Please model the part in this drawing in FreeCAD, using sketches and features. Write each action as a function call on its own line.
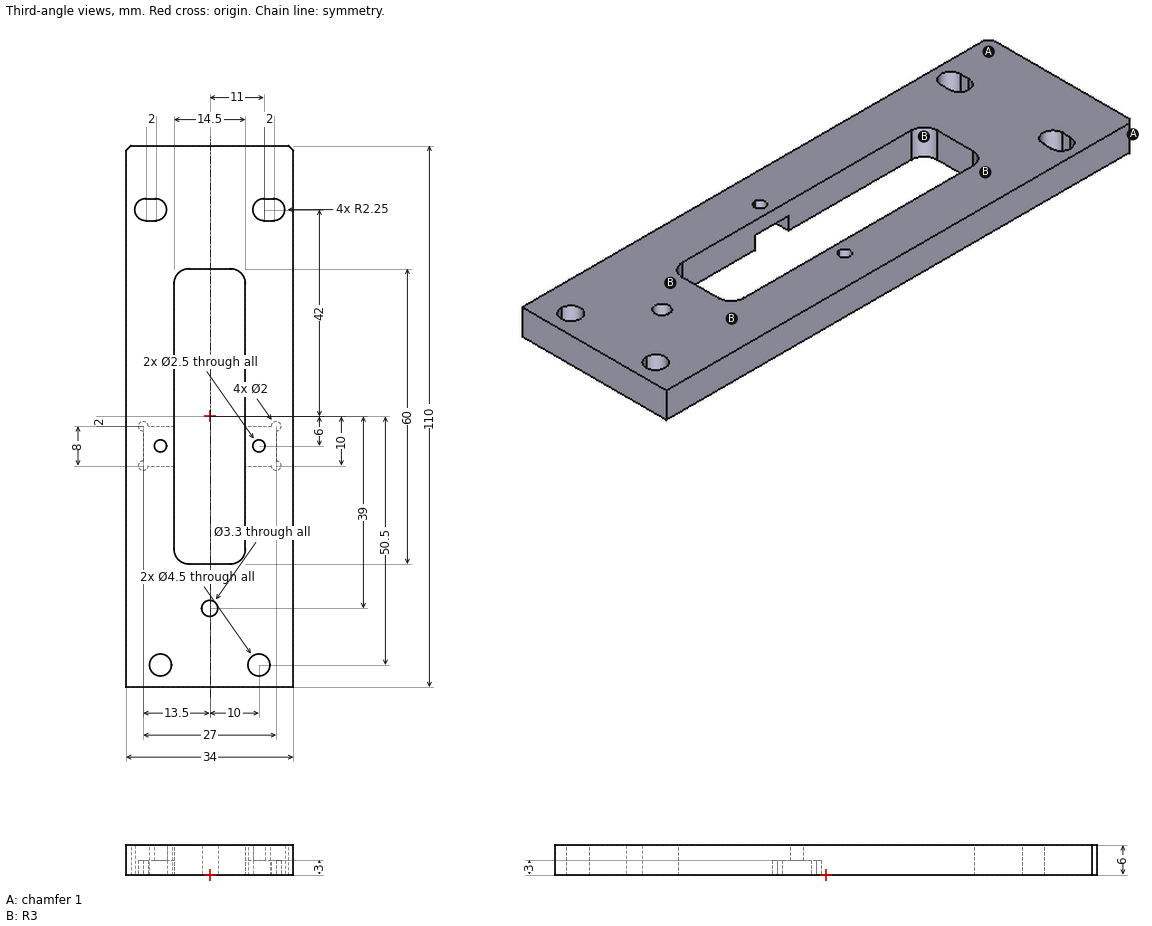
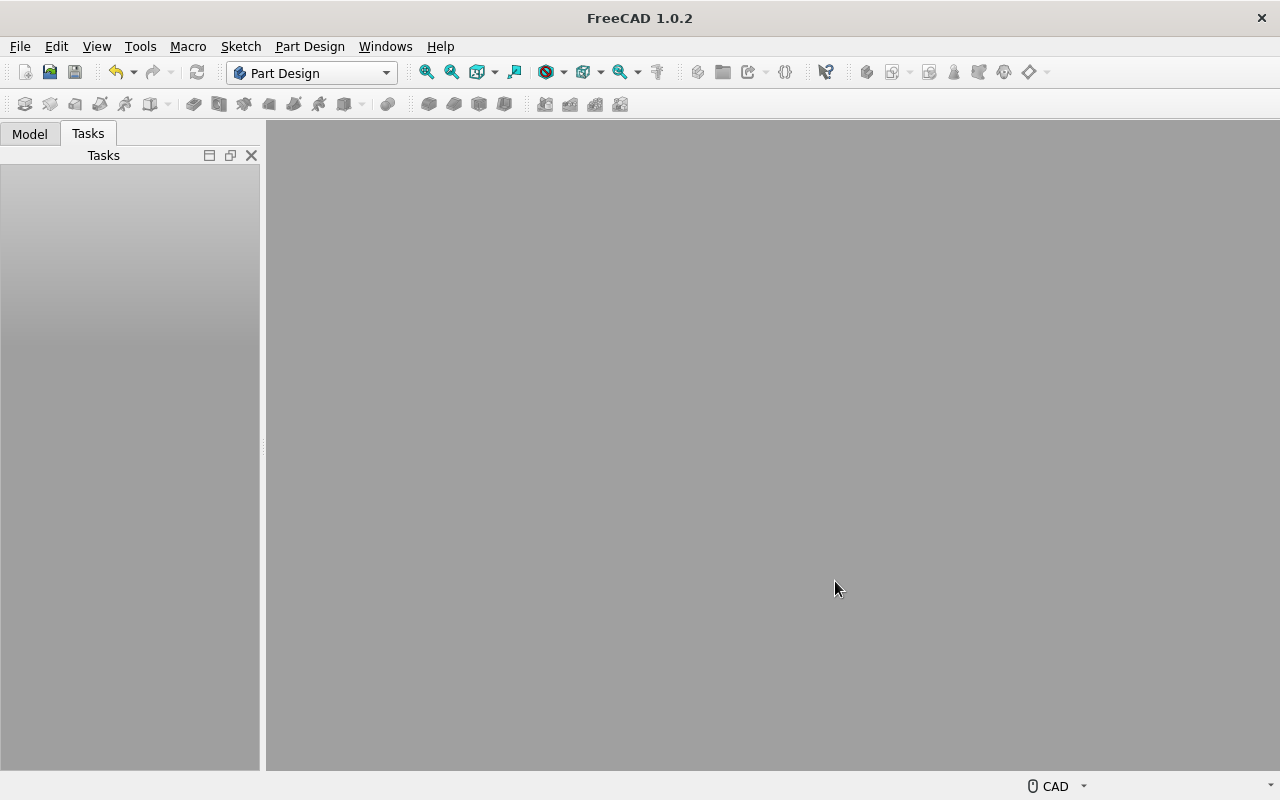
key(ctrl+n)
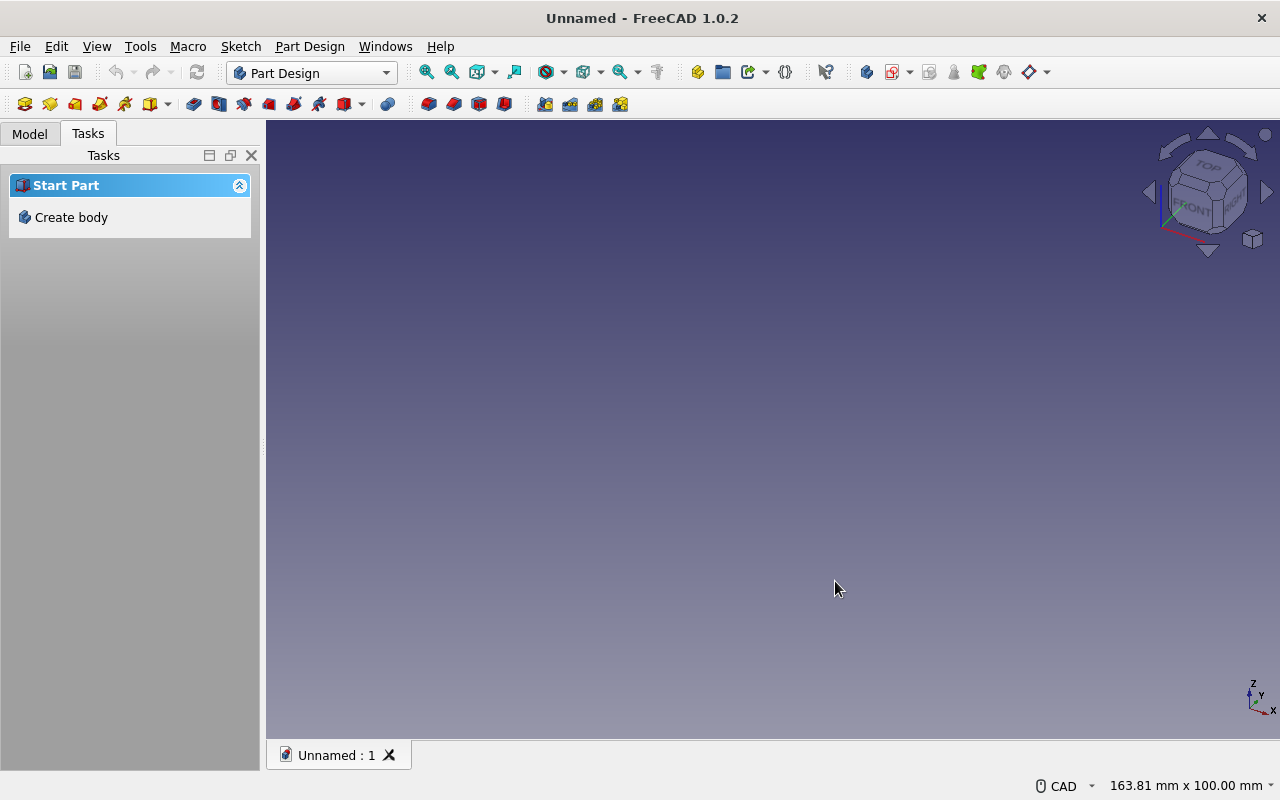
click(892, 72)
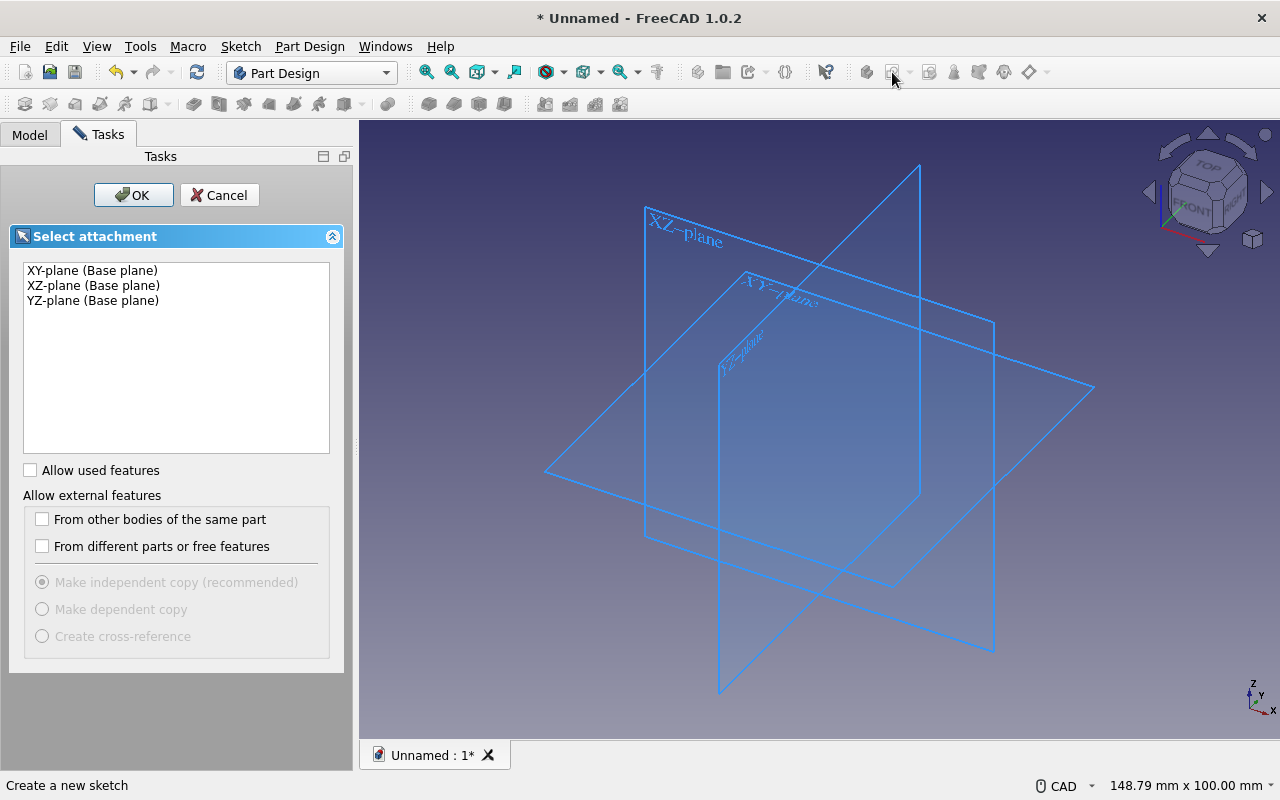
click(84, 270)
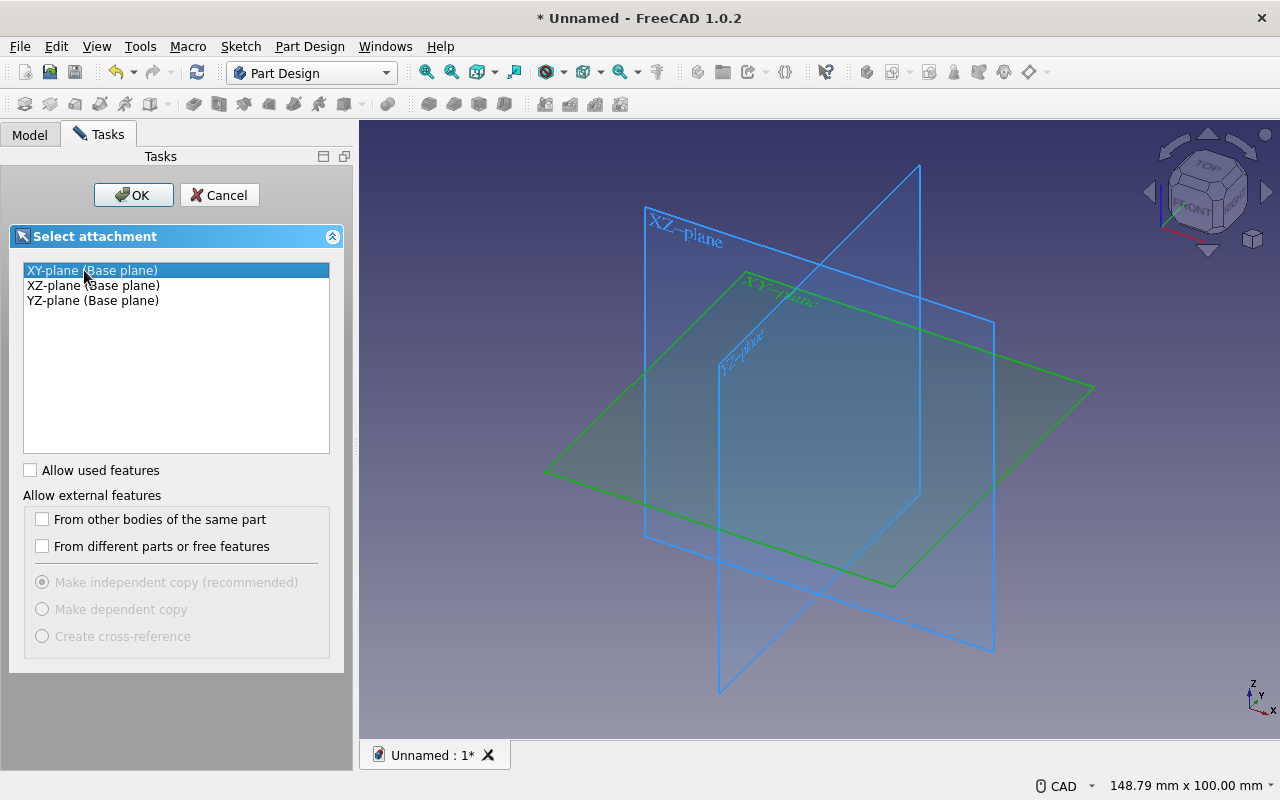
click(134, 195)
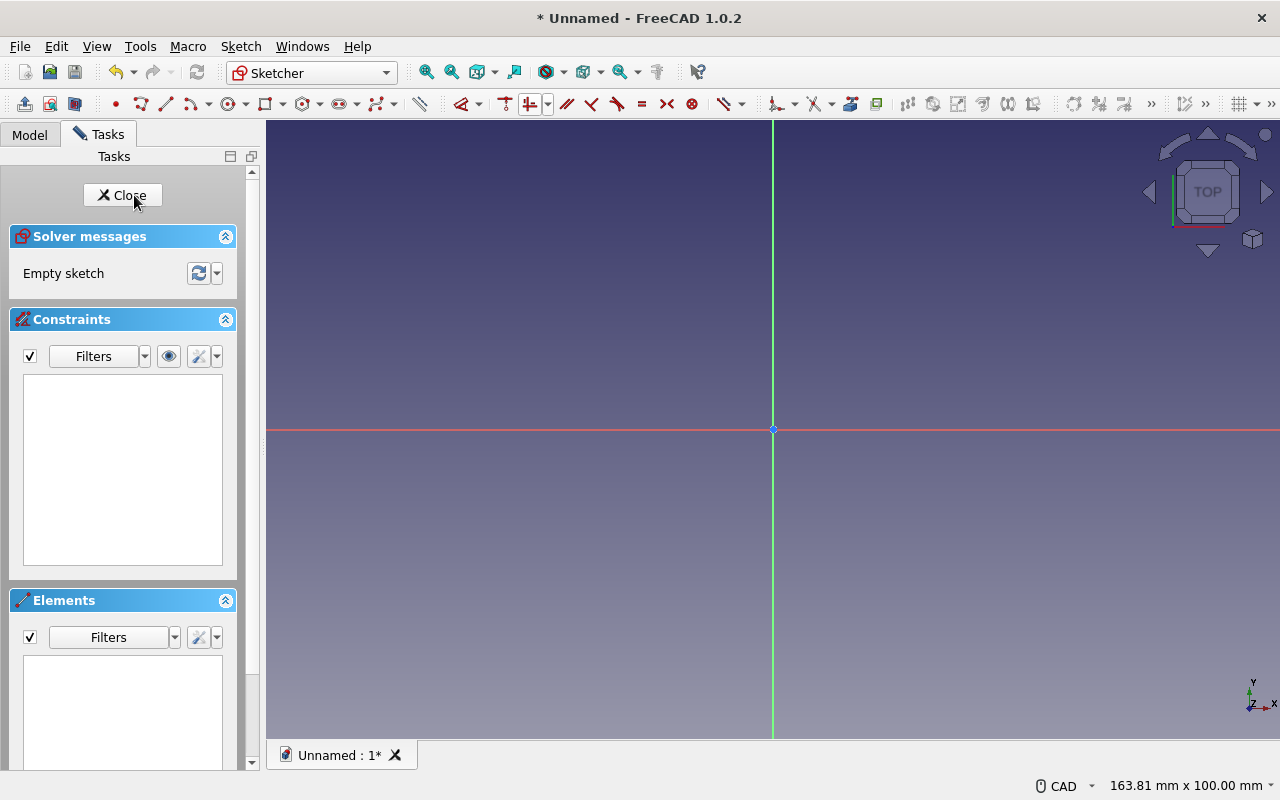
scroll(621, 430, down, 3)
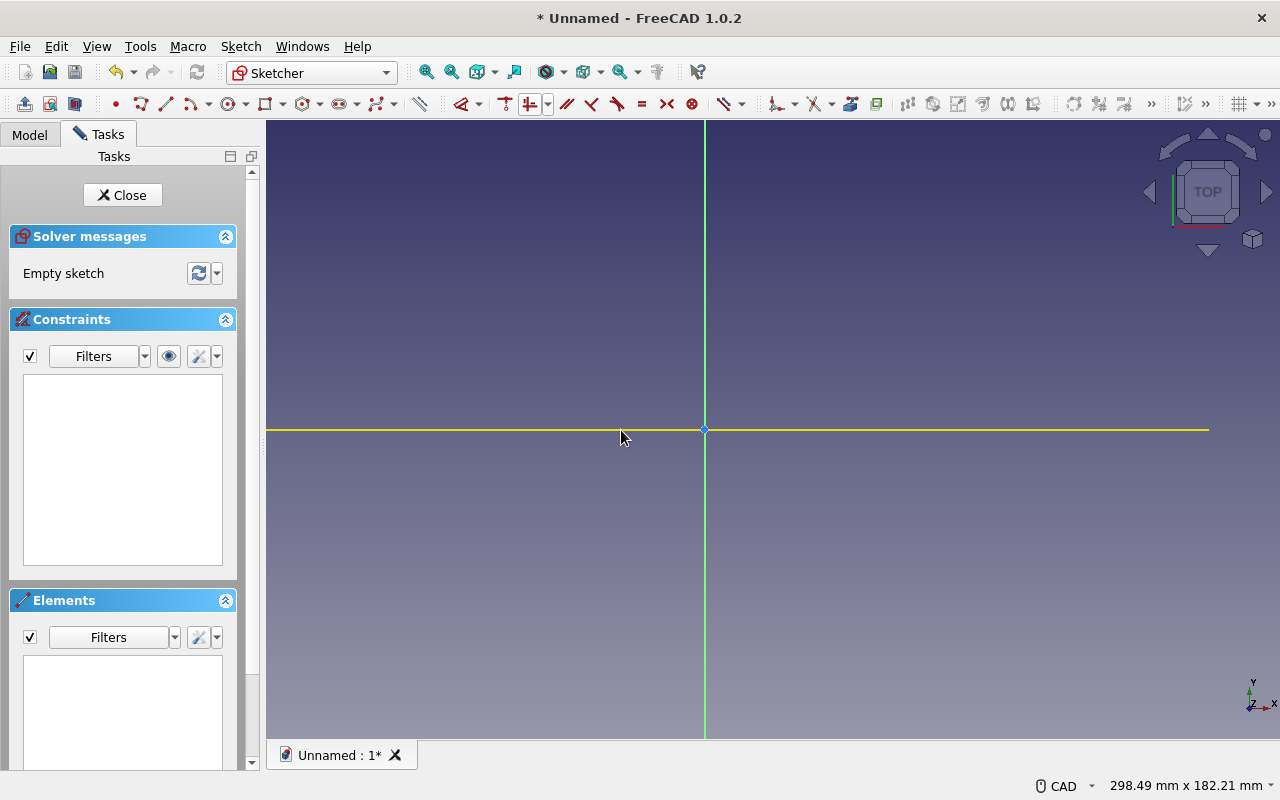
key(g)
key(v)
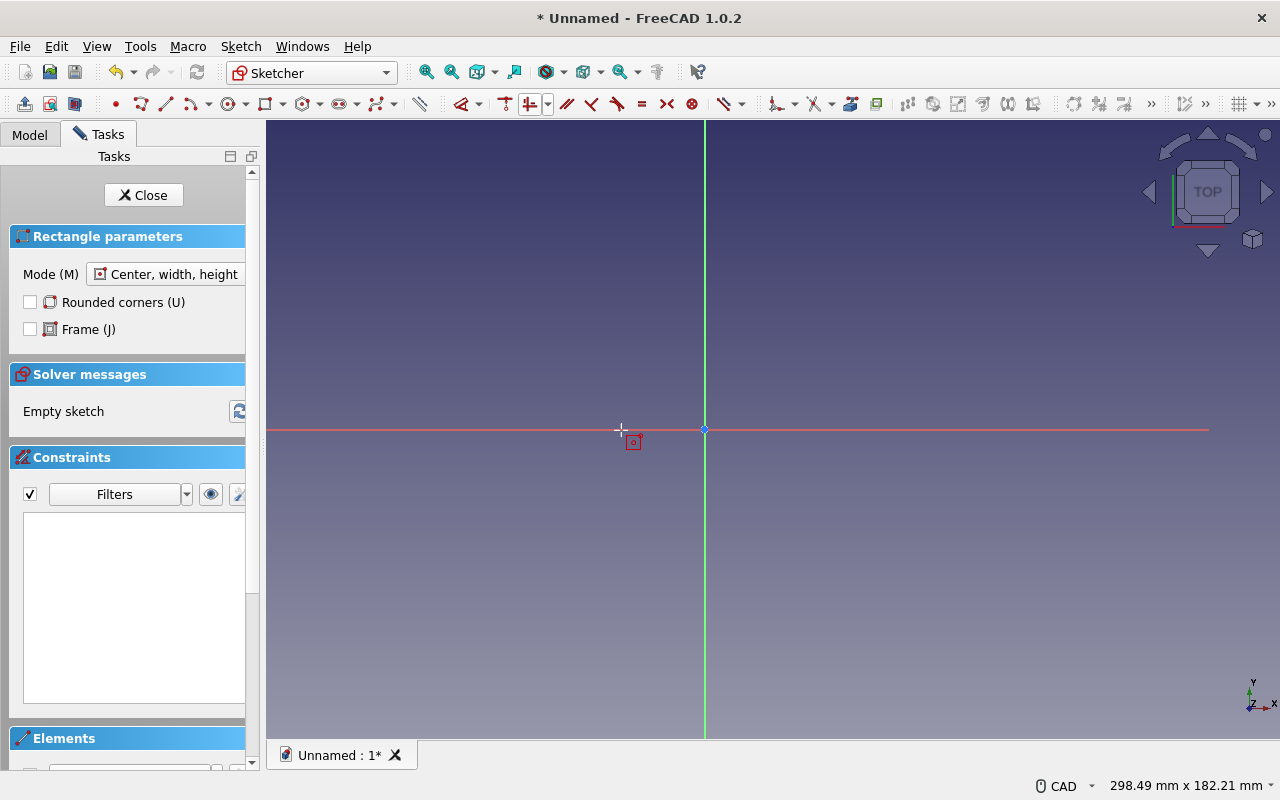
click(705, 430)
click(762, 243)
key(Escape)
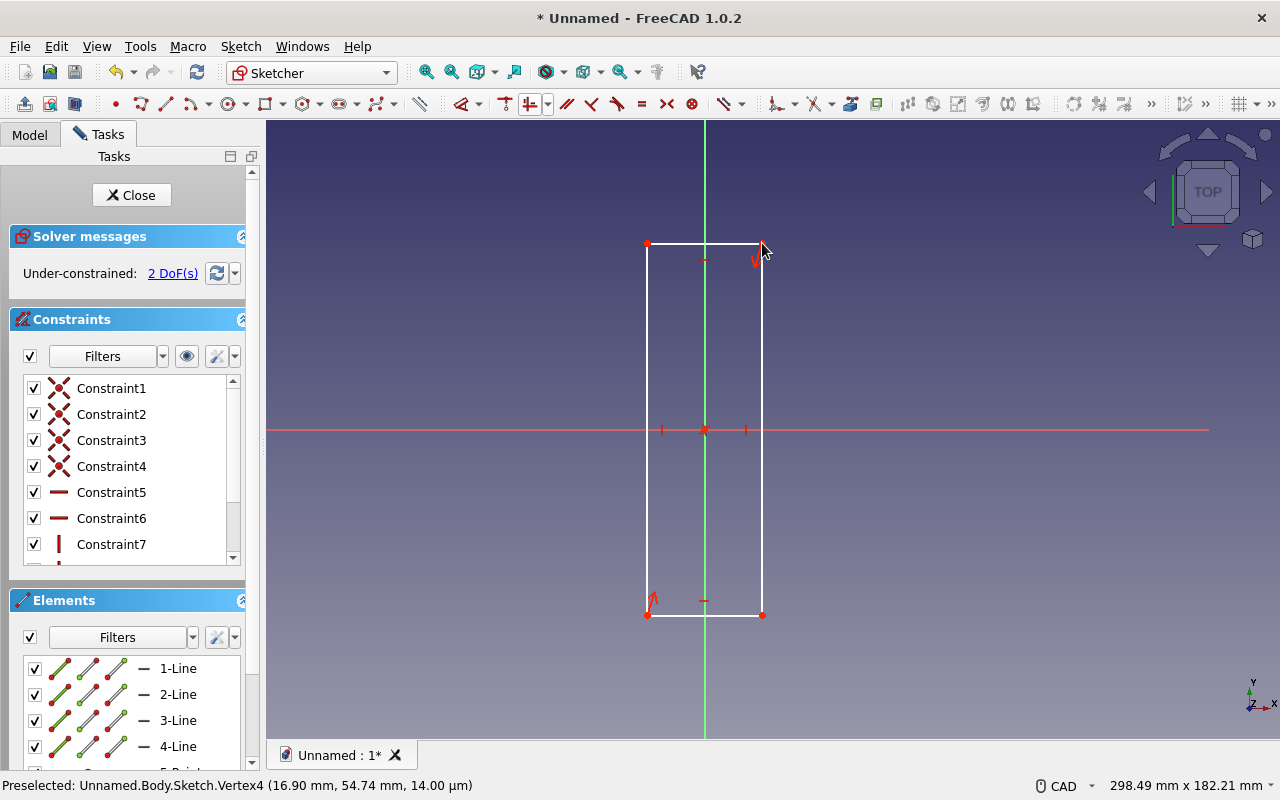
click(682, 616)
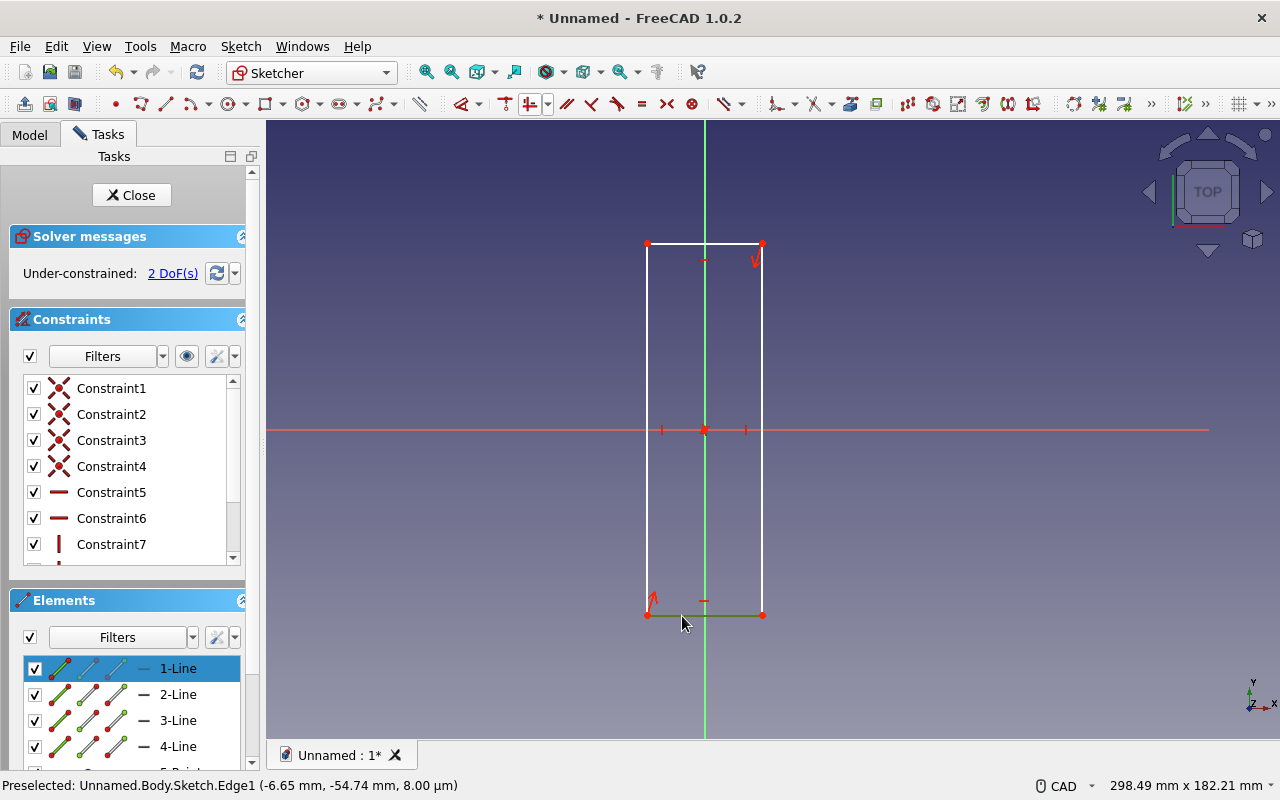
key(l)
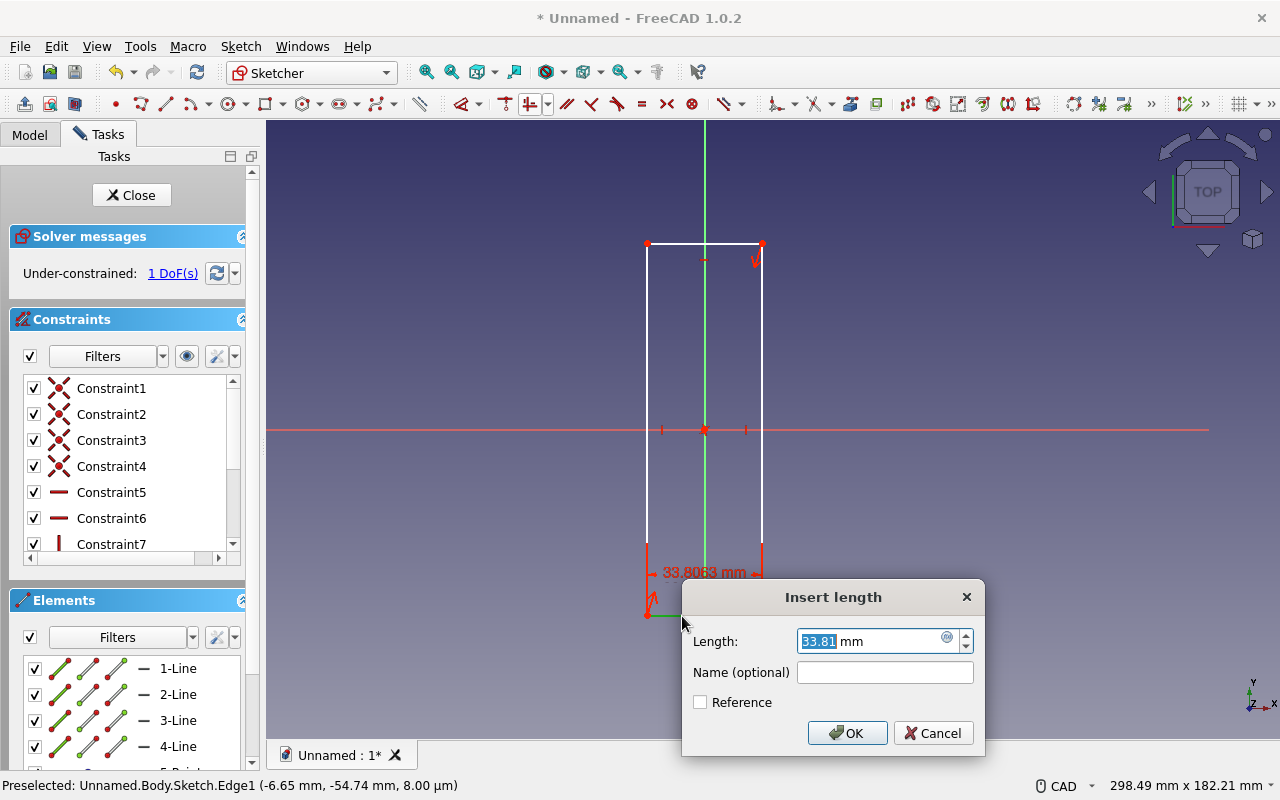
text(34)
key(Return)